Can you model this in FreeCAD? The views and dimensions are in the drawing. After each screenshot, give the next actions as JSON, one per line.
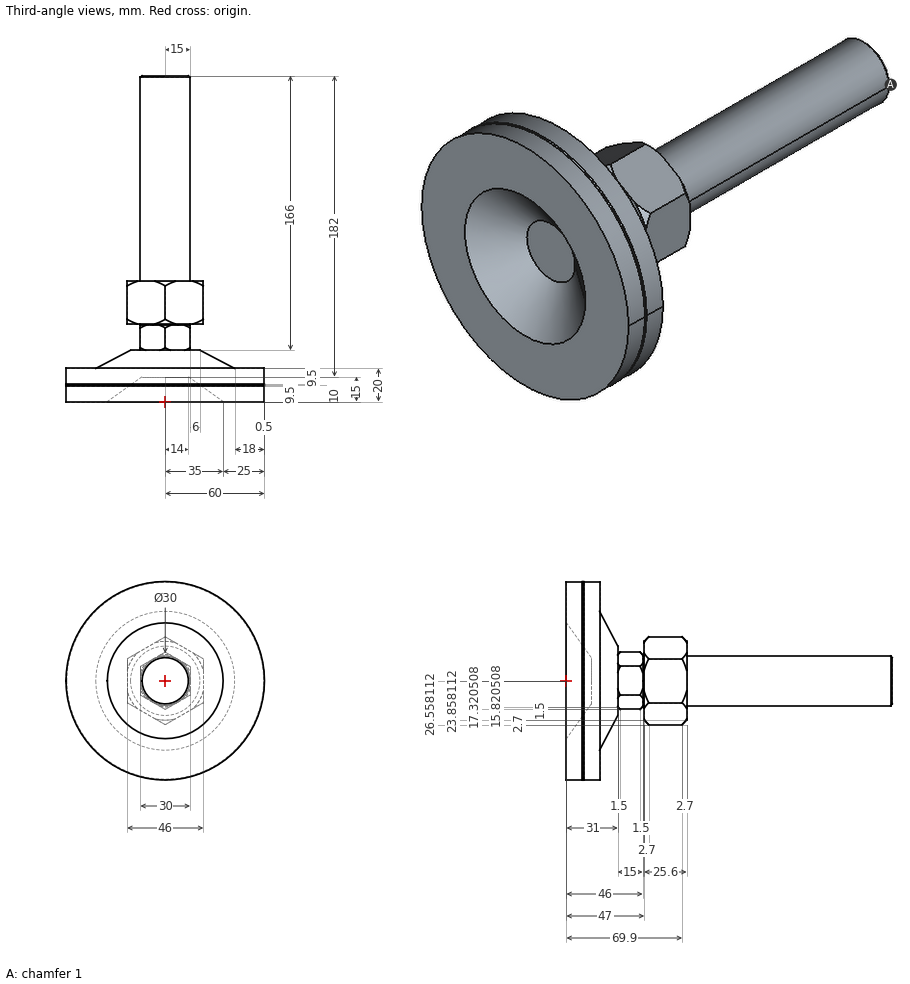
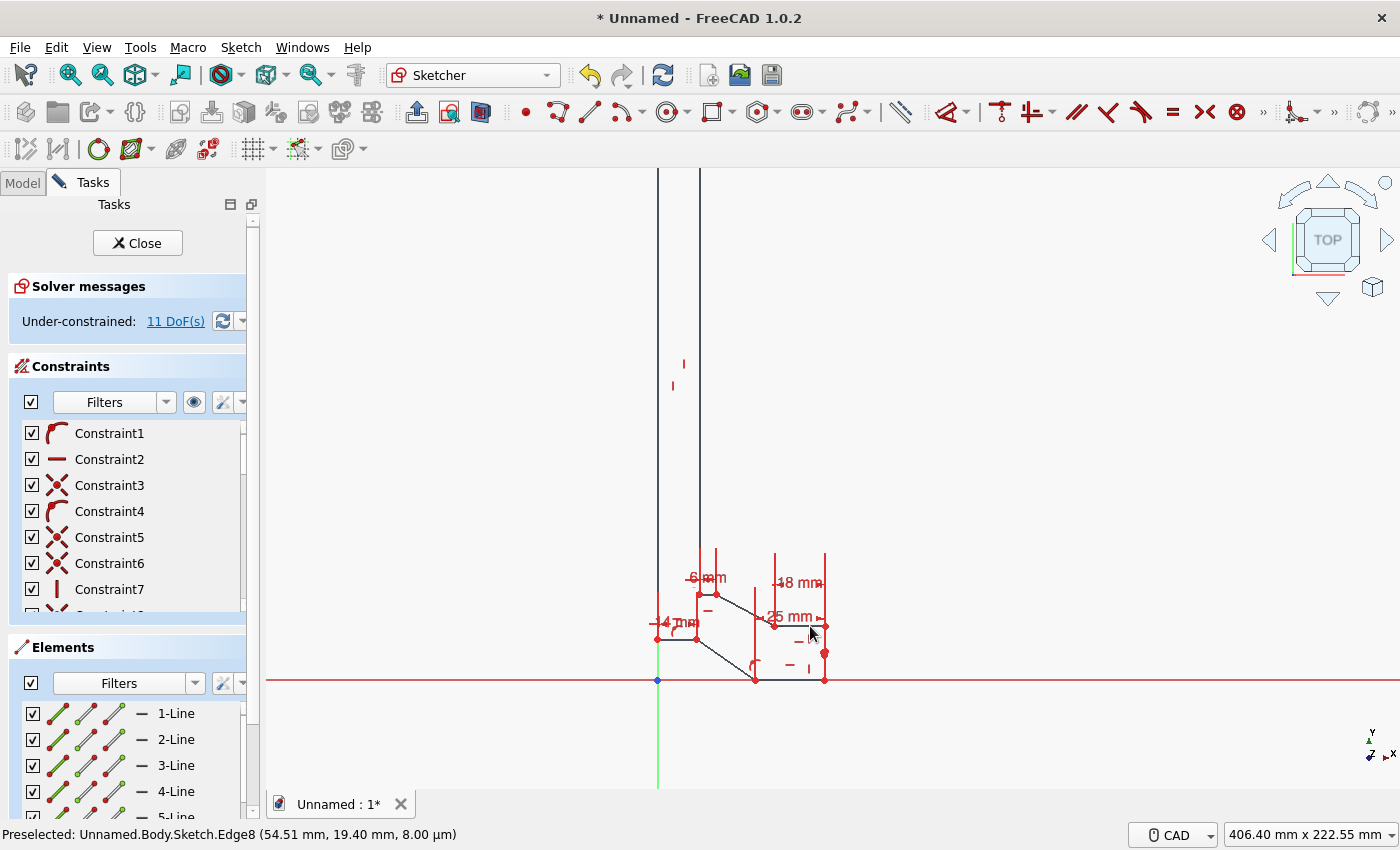
{"action": "scroll", "coordinate": [811, 627], "scroll_direction": "down", "scroll_amount": 2}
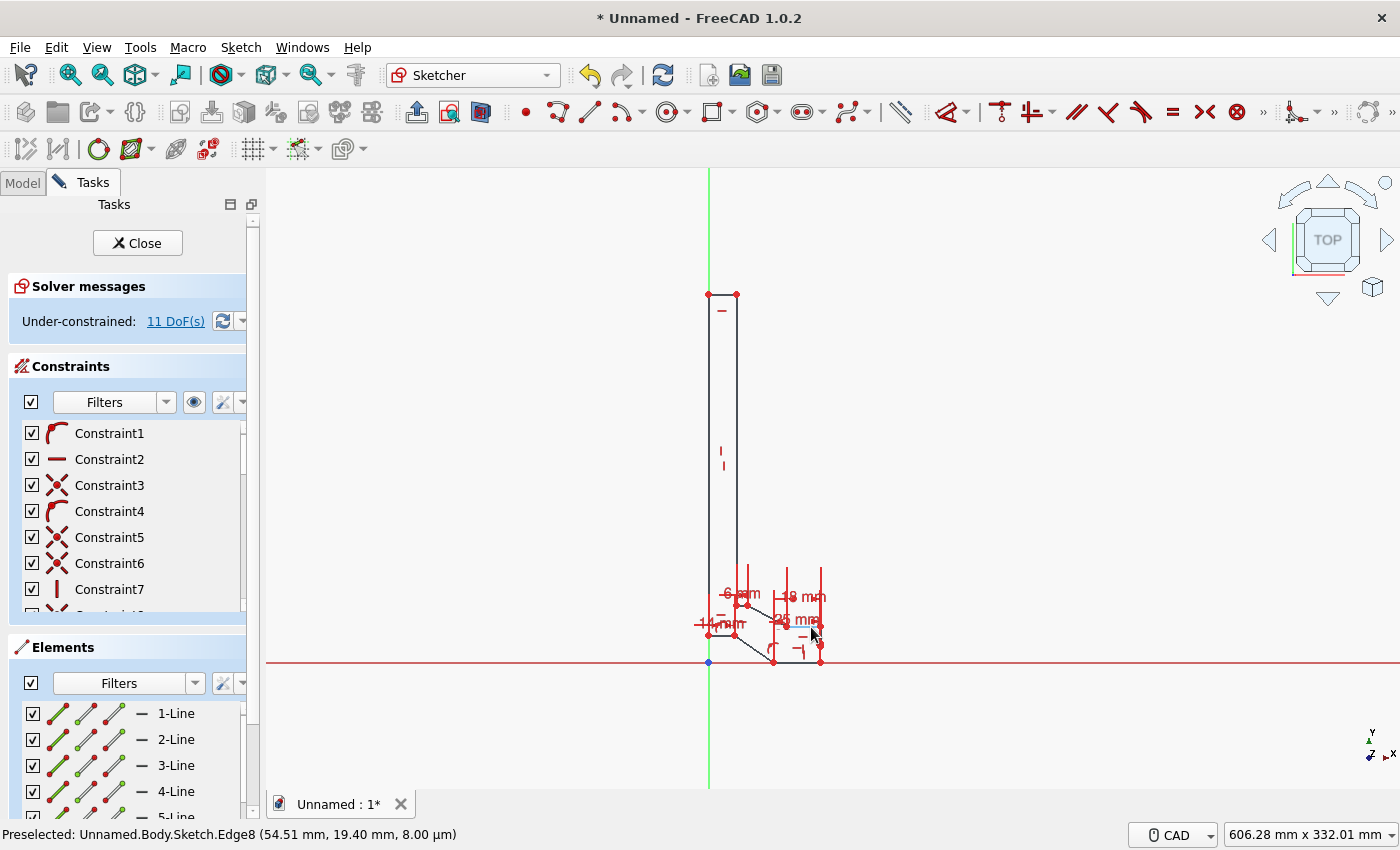
{"action": "scroll", "coordinate": [728, 295], "scroll_direction": "up", "scroll_amount": 3}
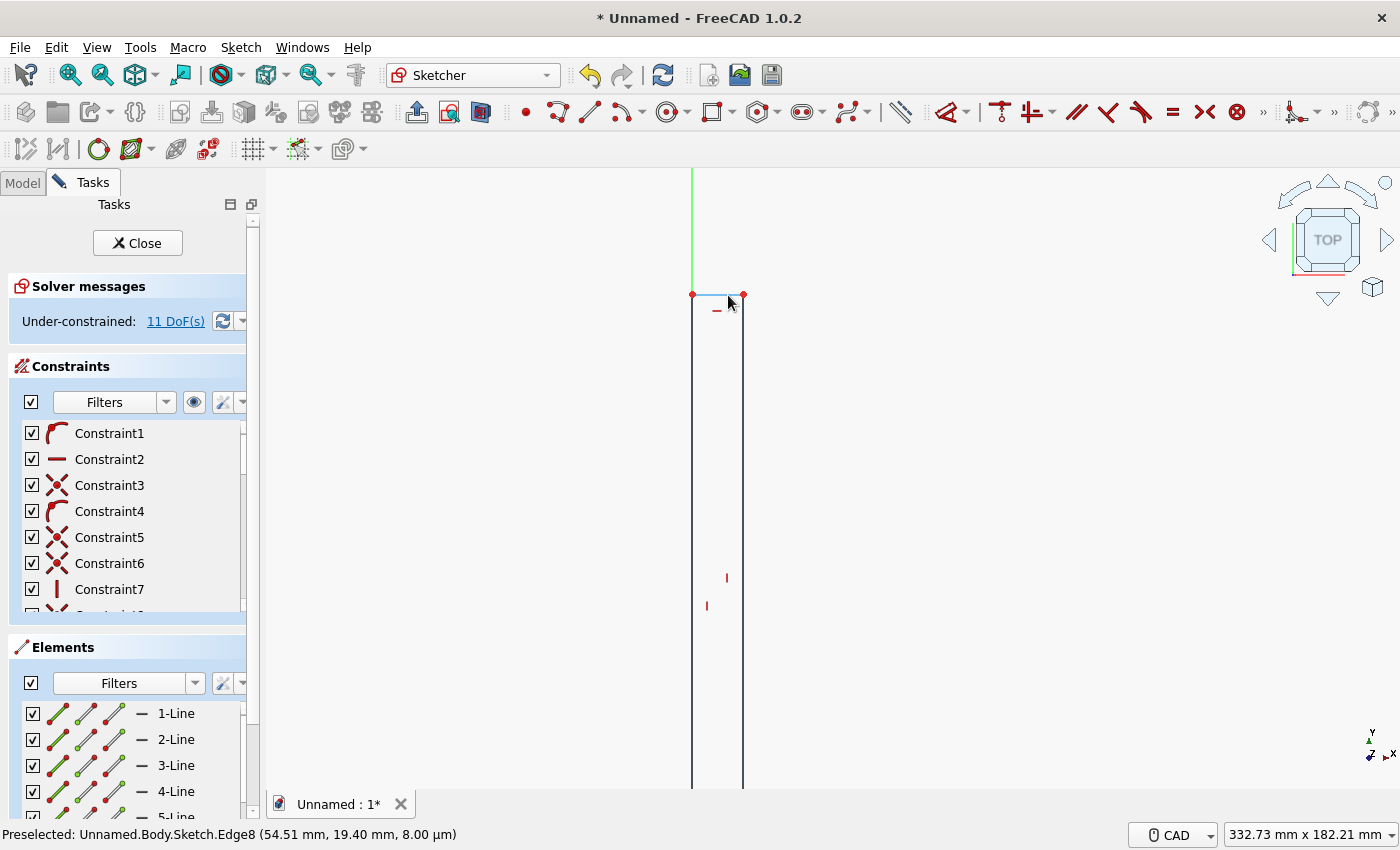
{"action": "left_click", "coordinate": [728, 295]}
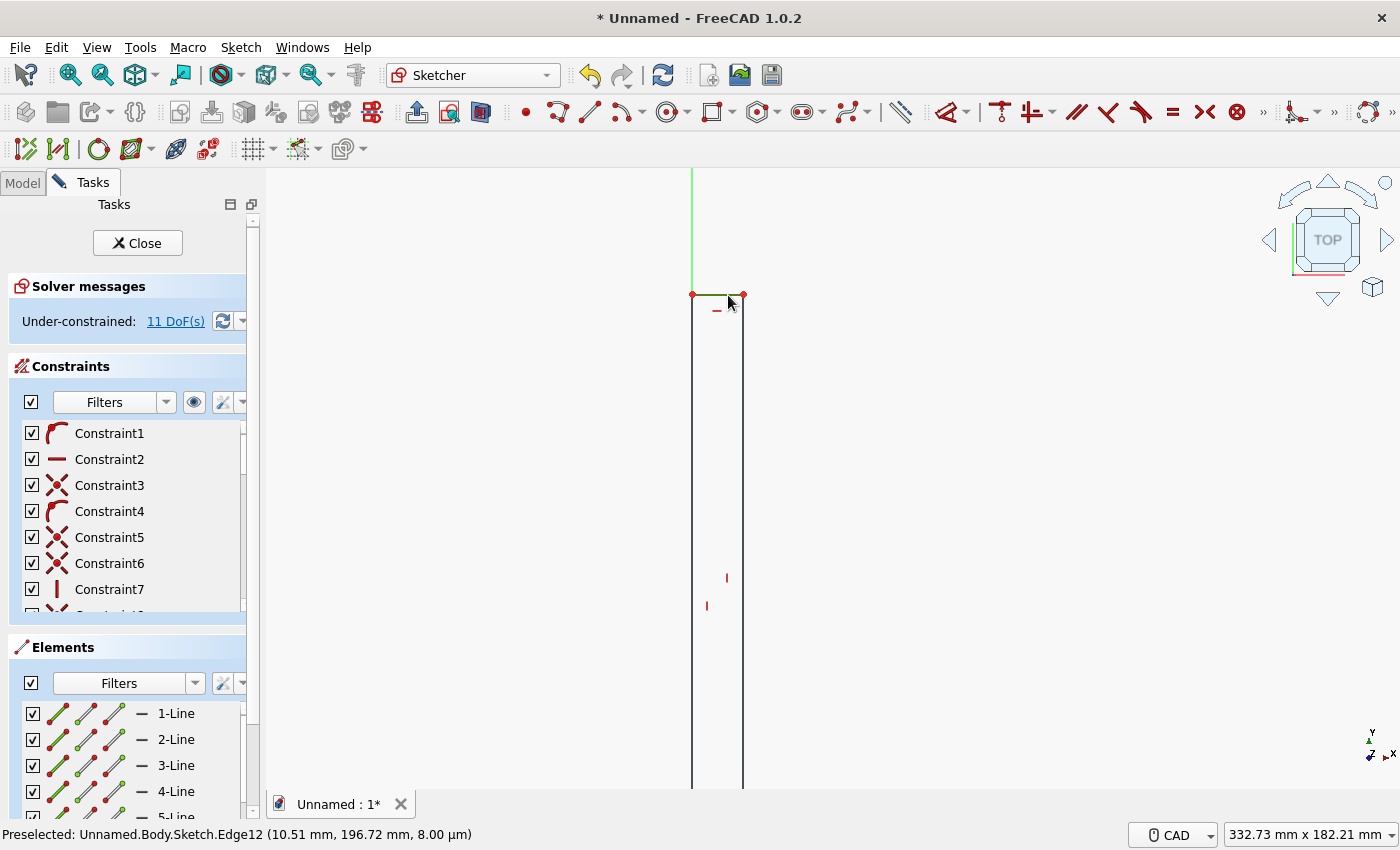
{"action": "key", "text": "l"}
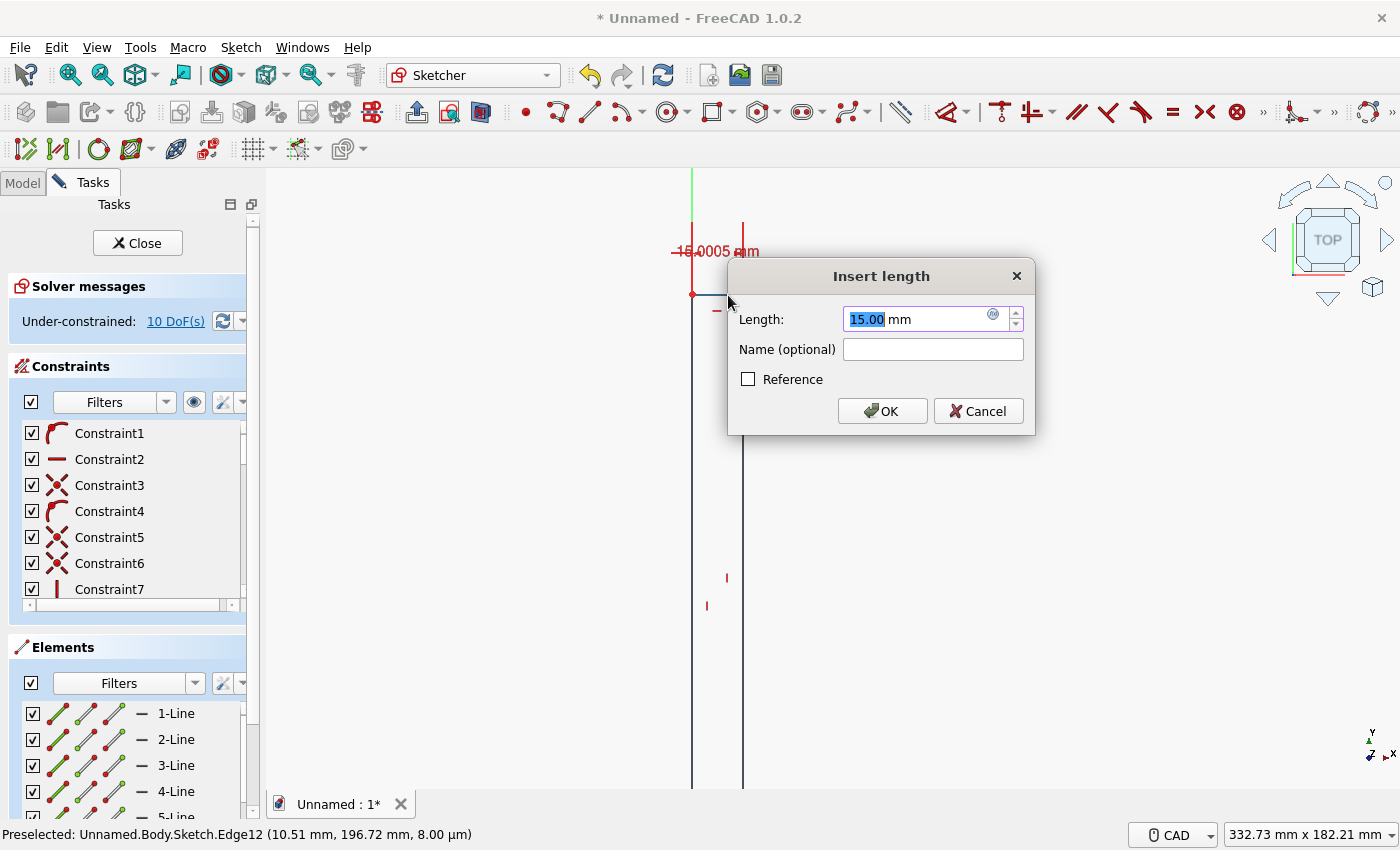
{"action": "type", "text": "15"}
{"action": "key", "text": "Return"}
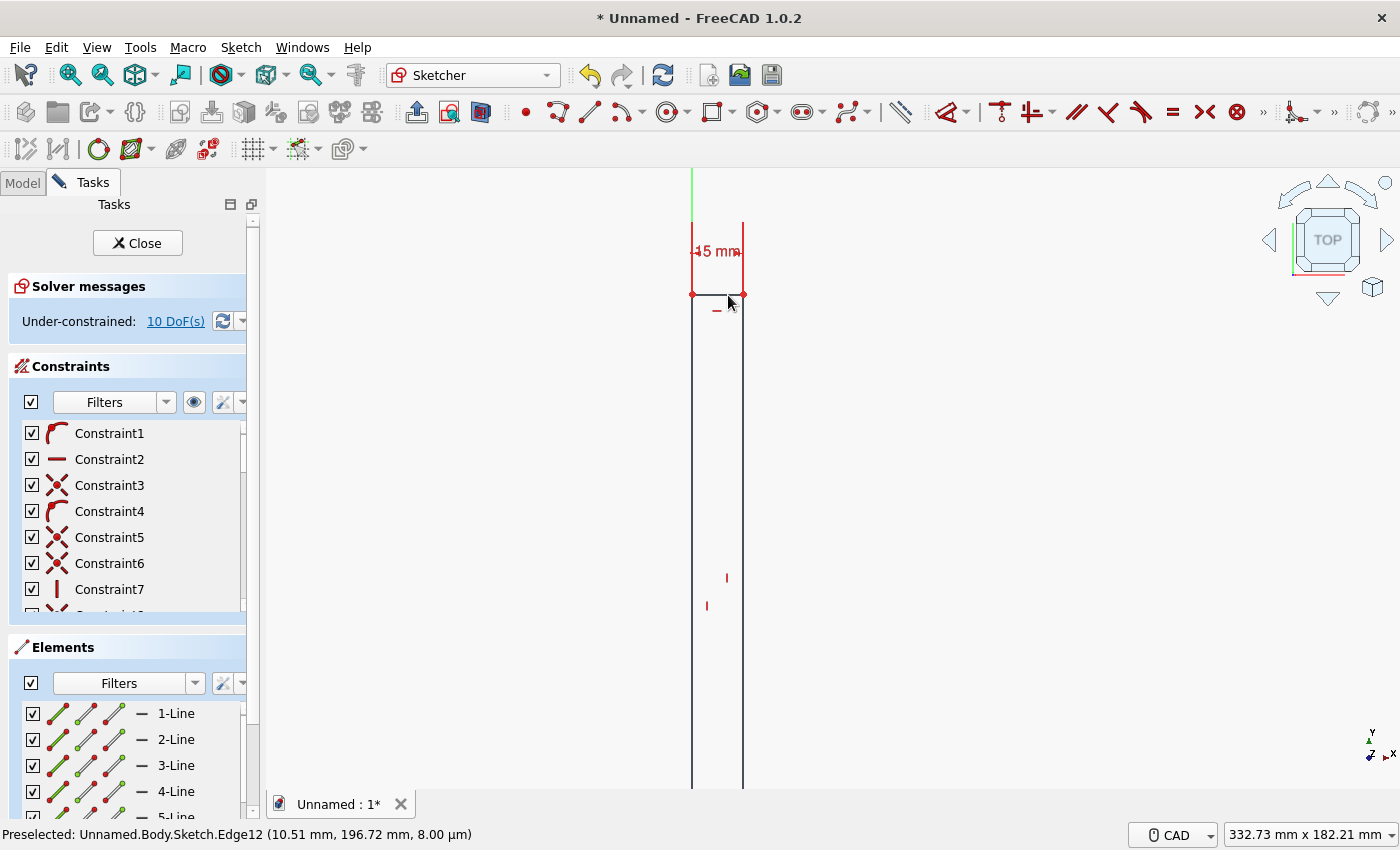
{"action": "scroll", "coordinate": [728, 295], "scroll_direction": "down", "scroll_amount": 3}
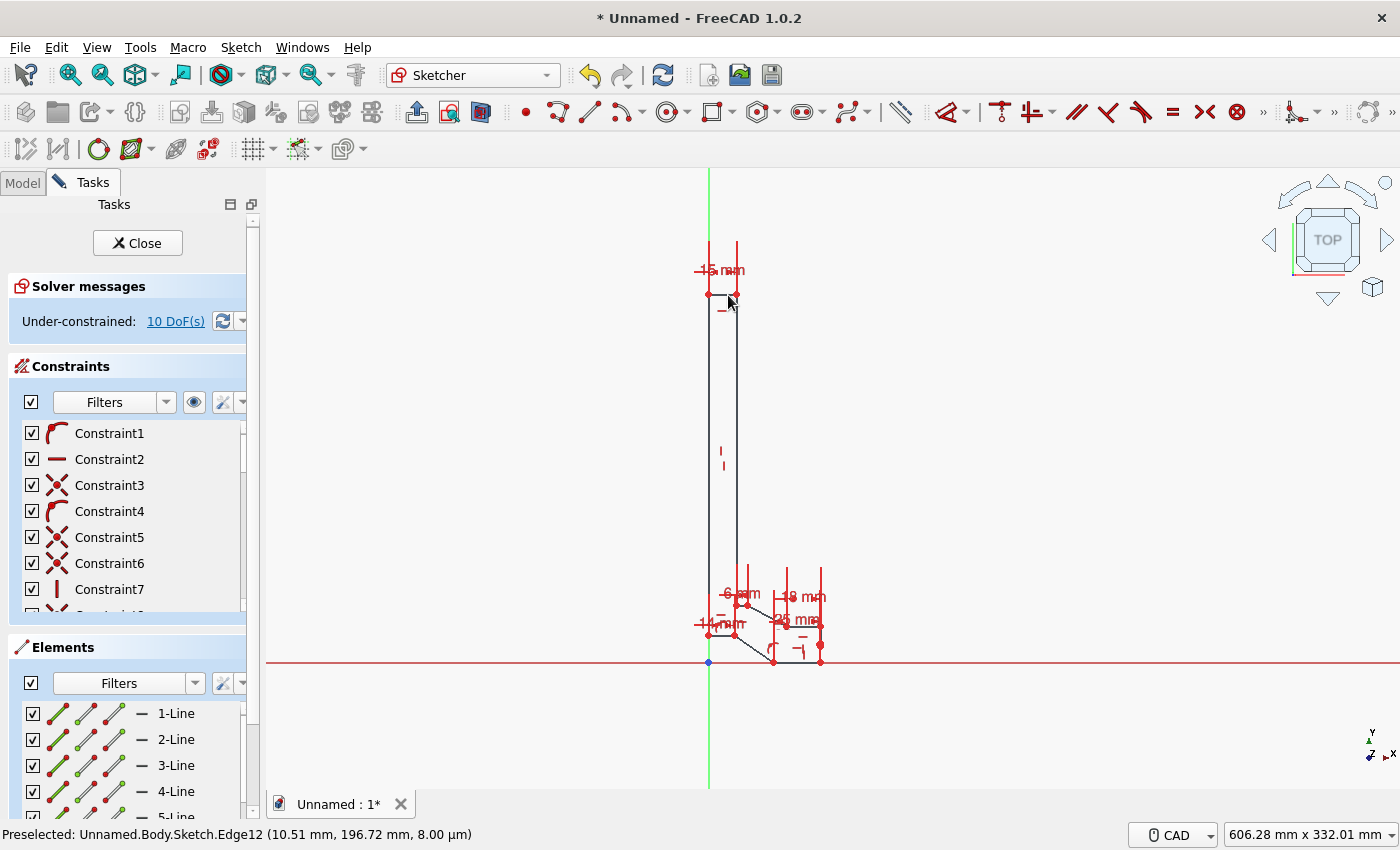
{"action": "scroll", "coordinate": [820, 656], "scroll_direction": "up", "scroll_amount": 5}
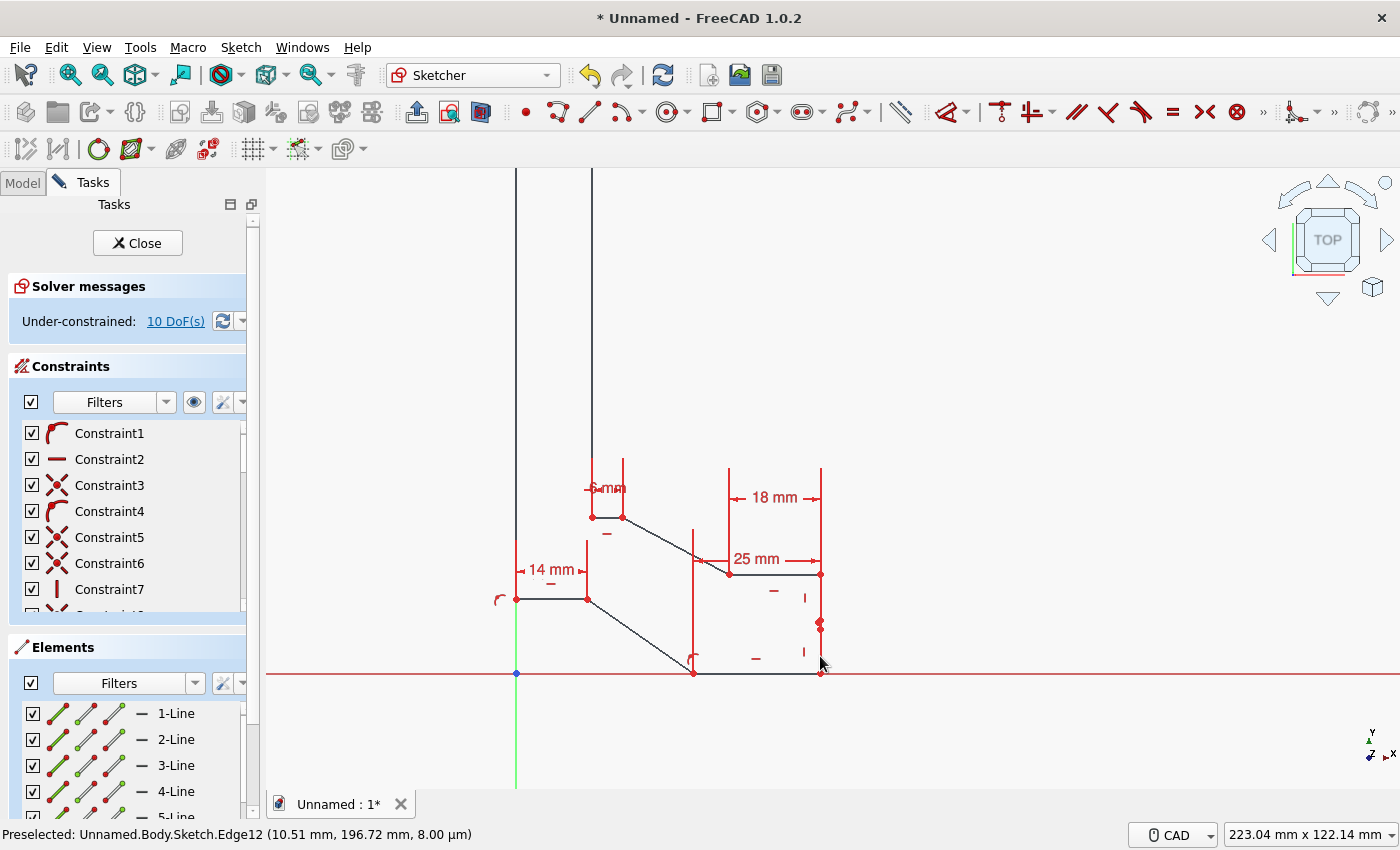
{"action": "left_click", "coordinate": [821, 656]}